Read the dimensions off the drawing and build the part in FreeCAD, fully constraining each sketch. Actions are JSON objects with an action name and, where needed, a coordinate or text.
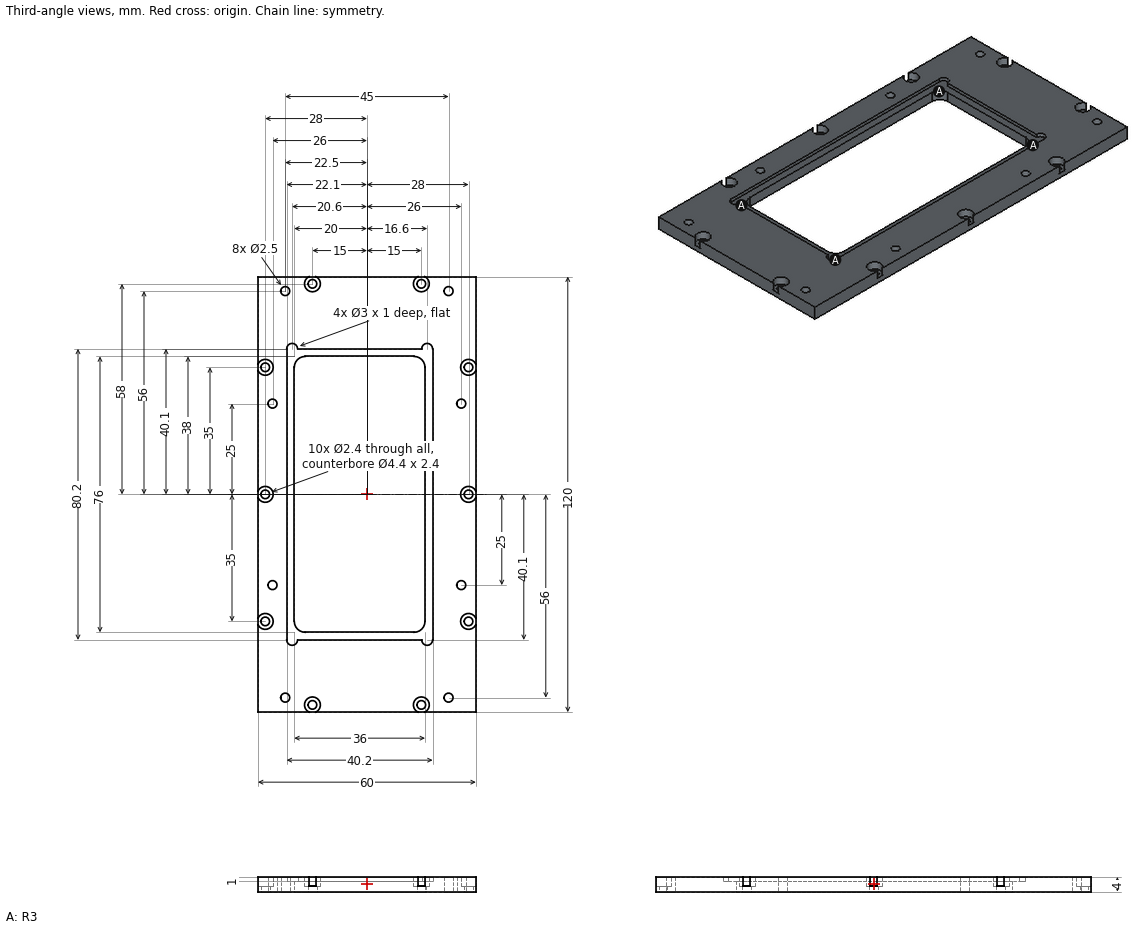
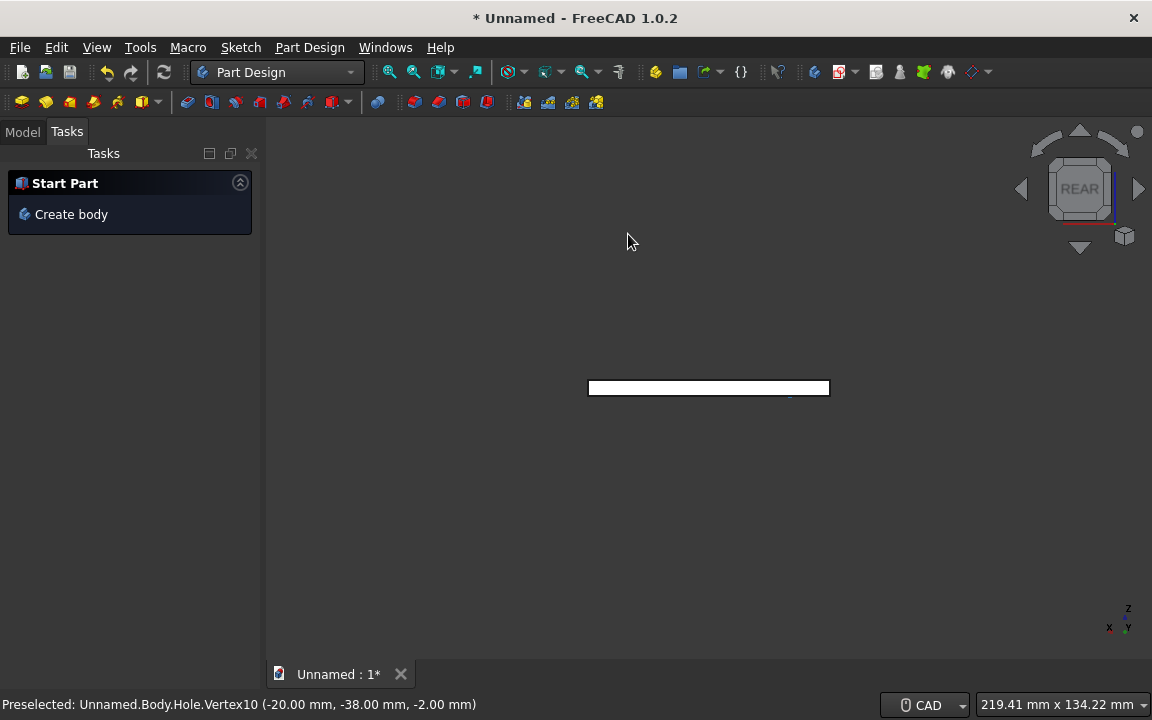
{"action": "key", "text": "v f"}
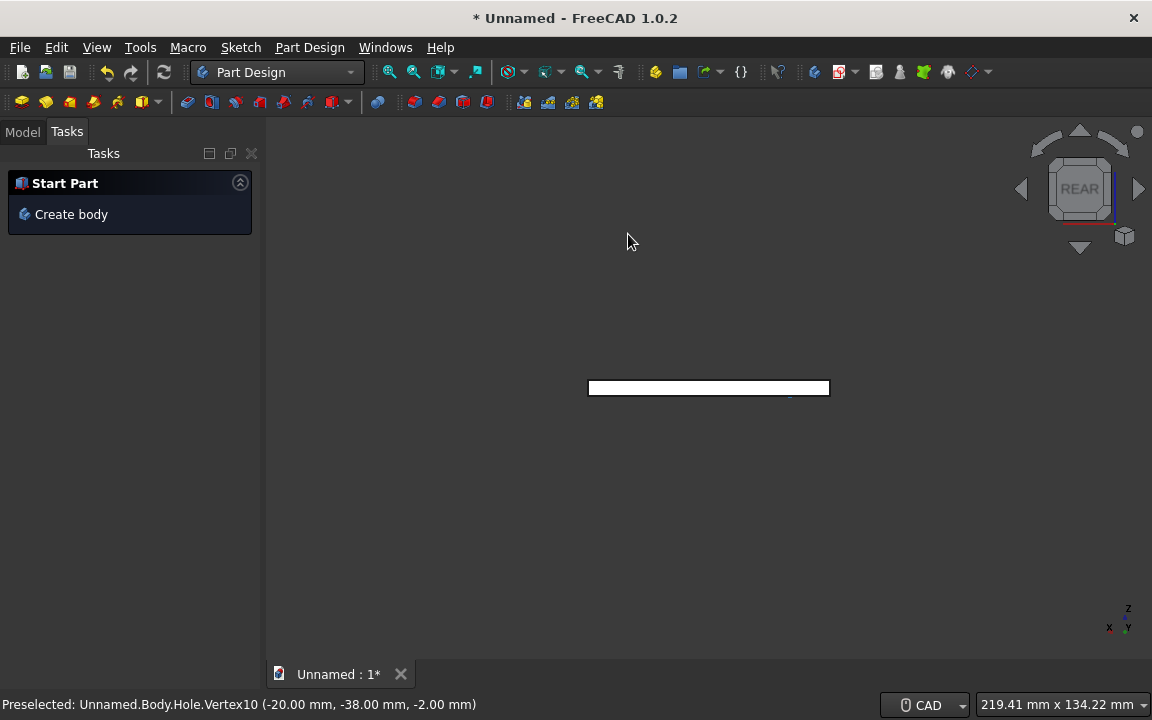
{"action": "scroll", "coordinate": [790, 389], "scroll_direction": "up", "scroll_amount": 6}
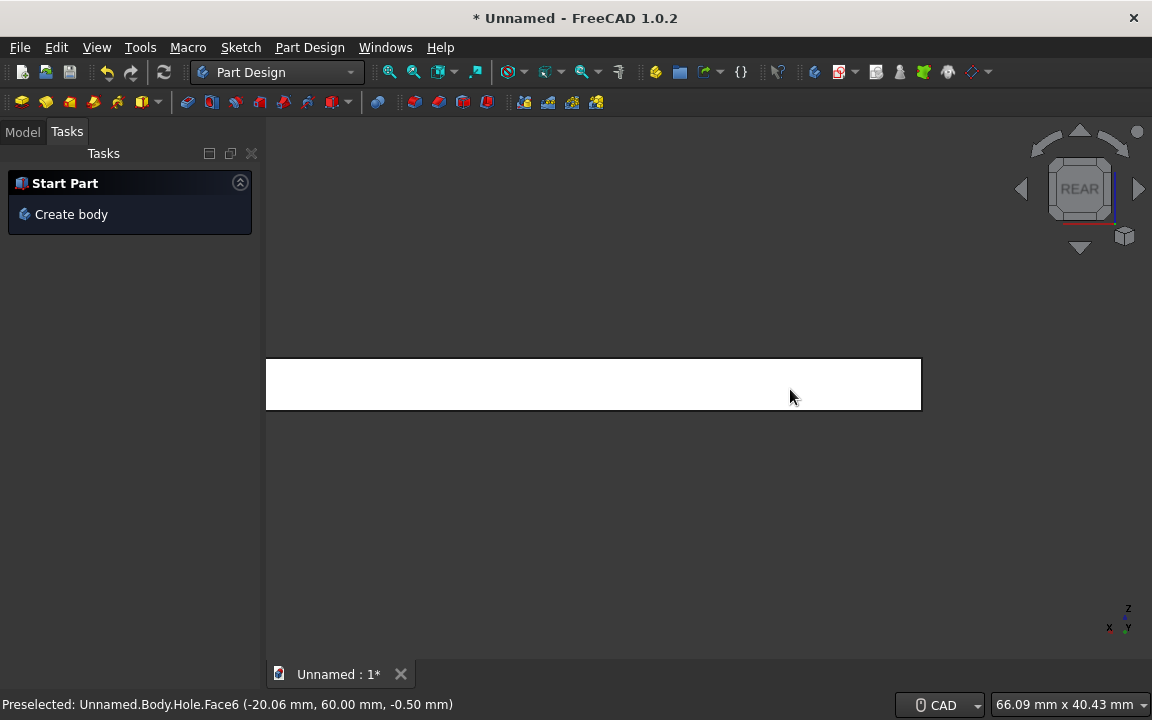
{"action": "key", "text": "v f"}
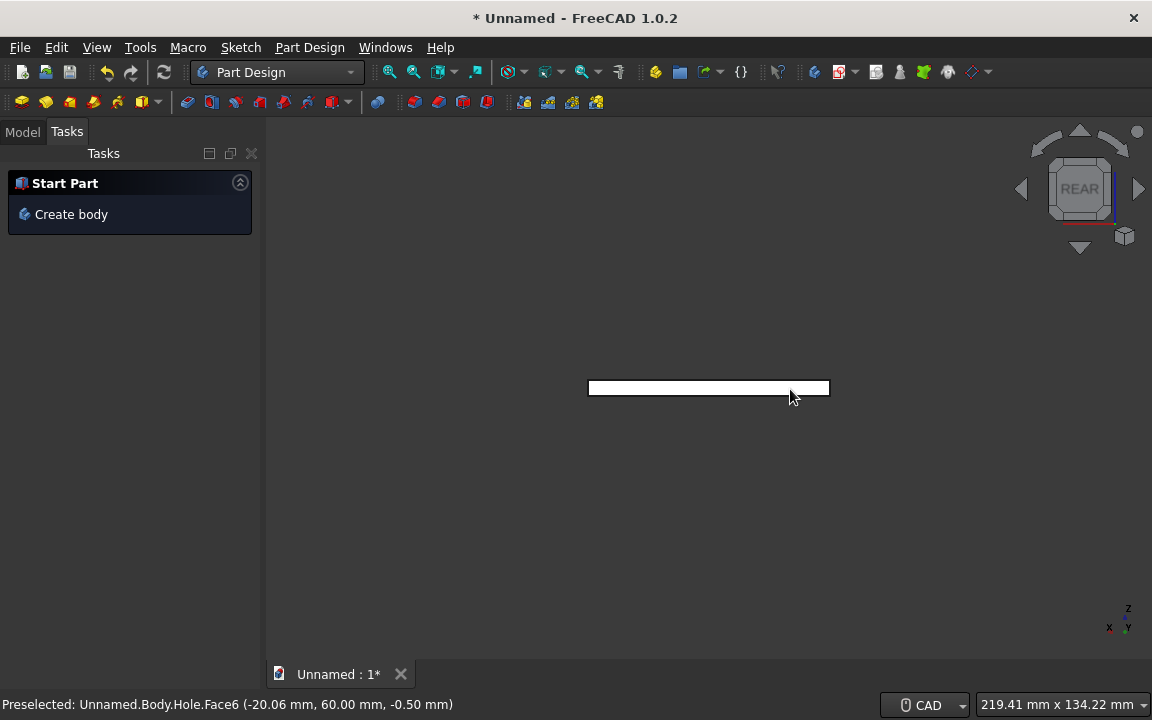
{"action": "key", "text": "6"}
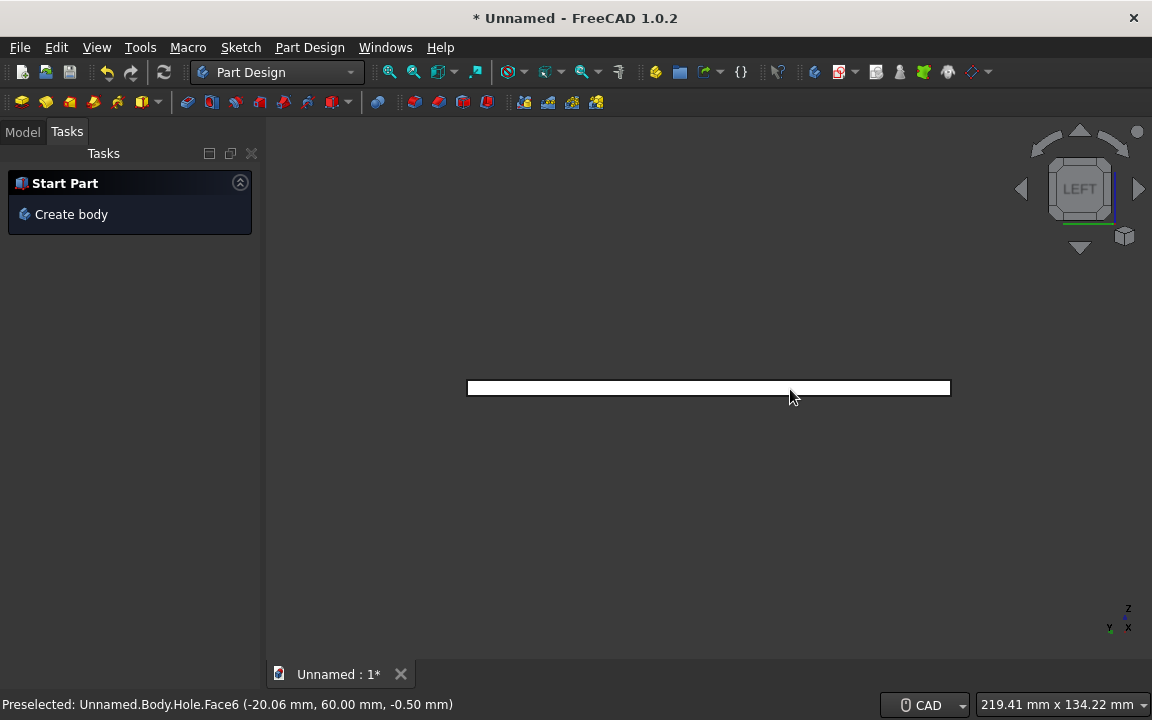
{"action": "scroll", "coordinate": [862, 389], "scroll_direction": "up", "scroll_amount": 6}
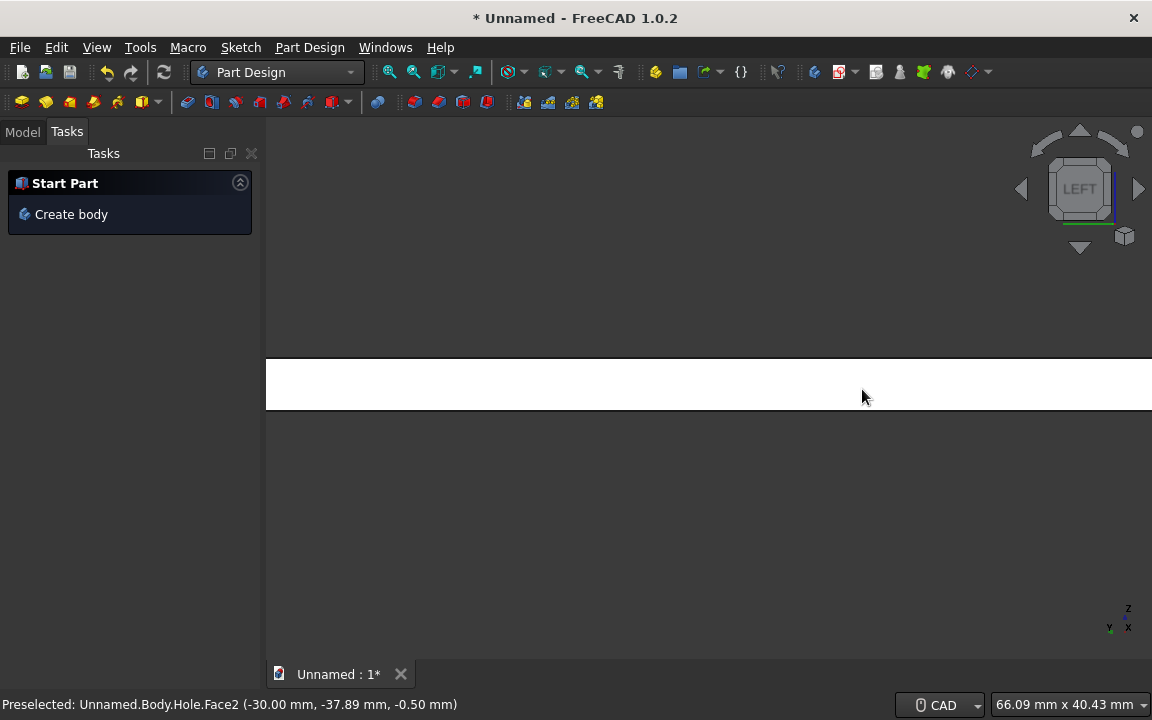
{"action": "key", "text": "v f"}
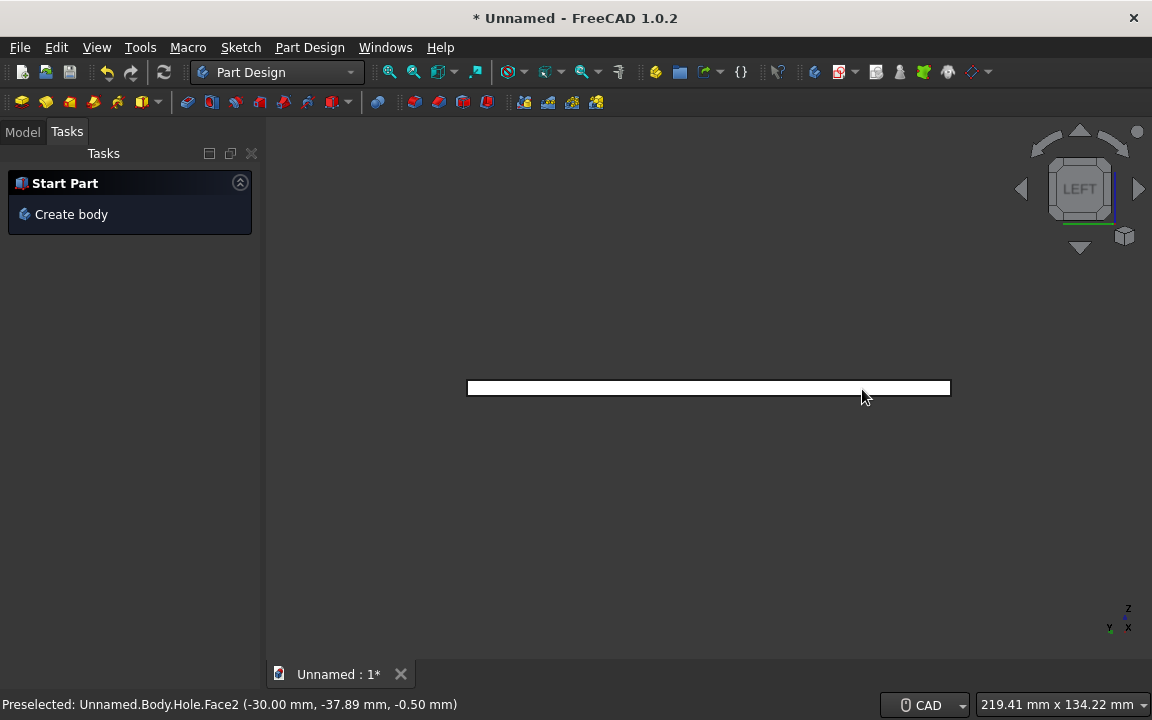
{"action": "key", "text": "v 3"}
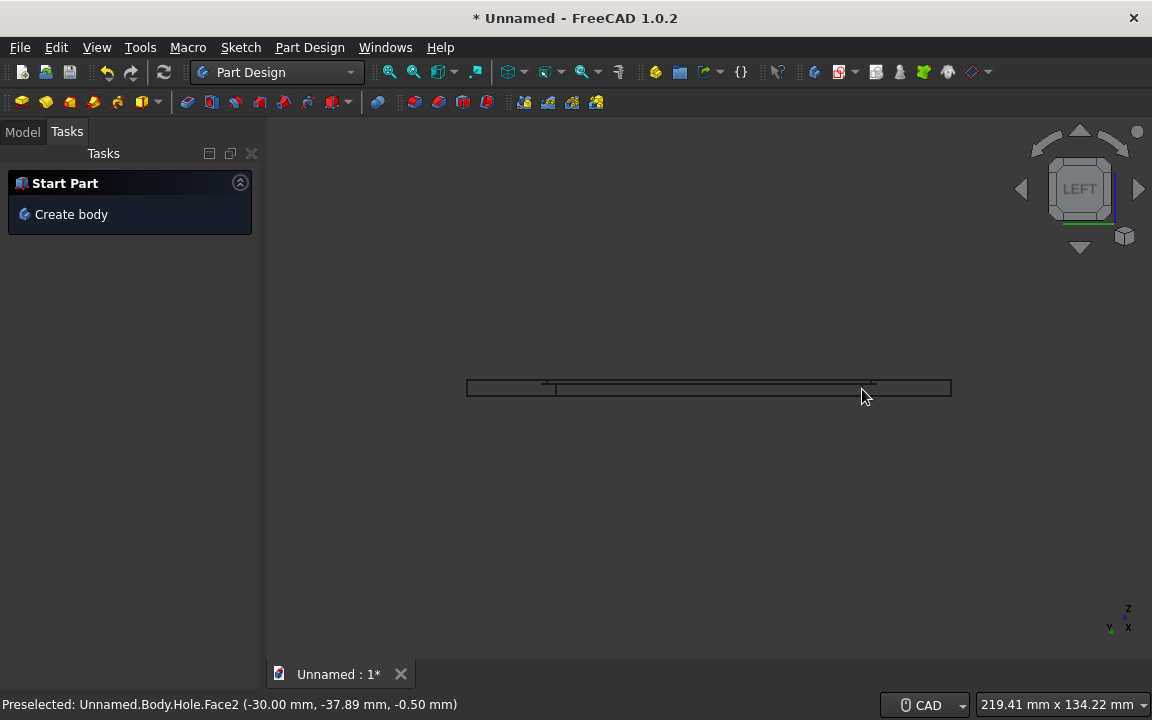
{"action": "key", "text": "0"}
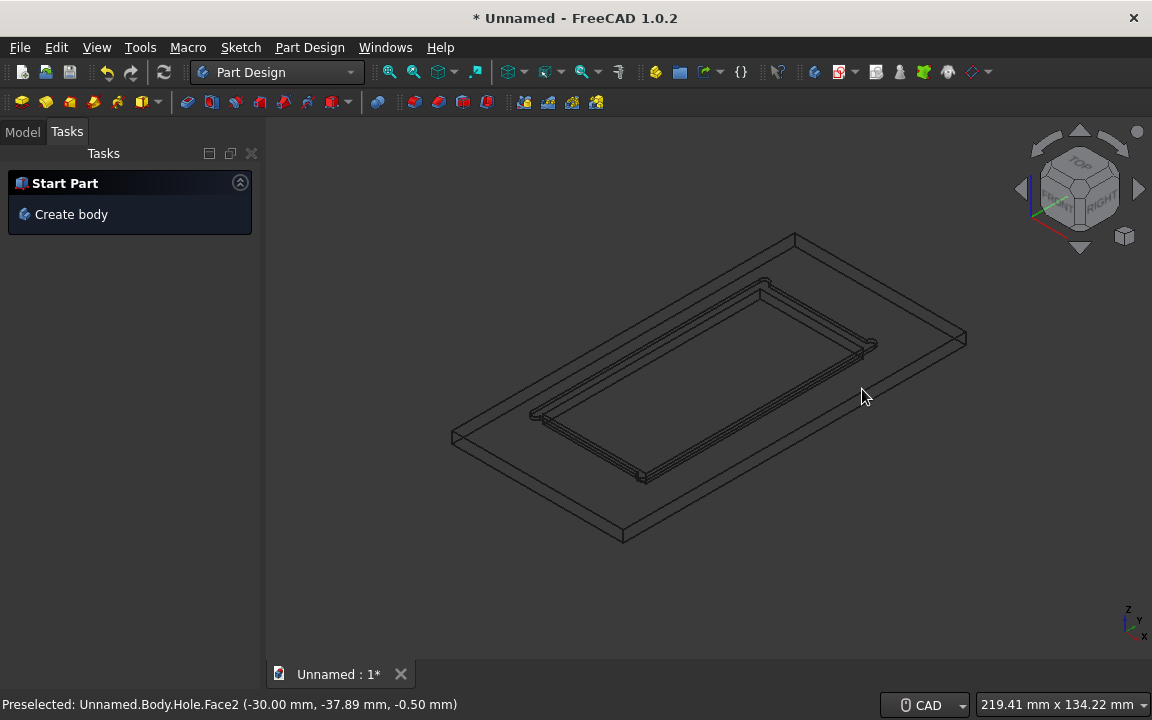
{"action": "left_click", "coordinate": [760, 296]}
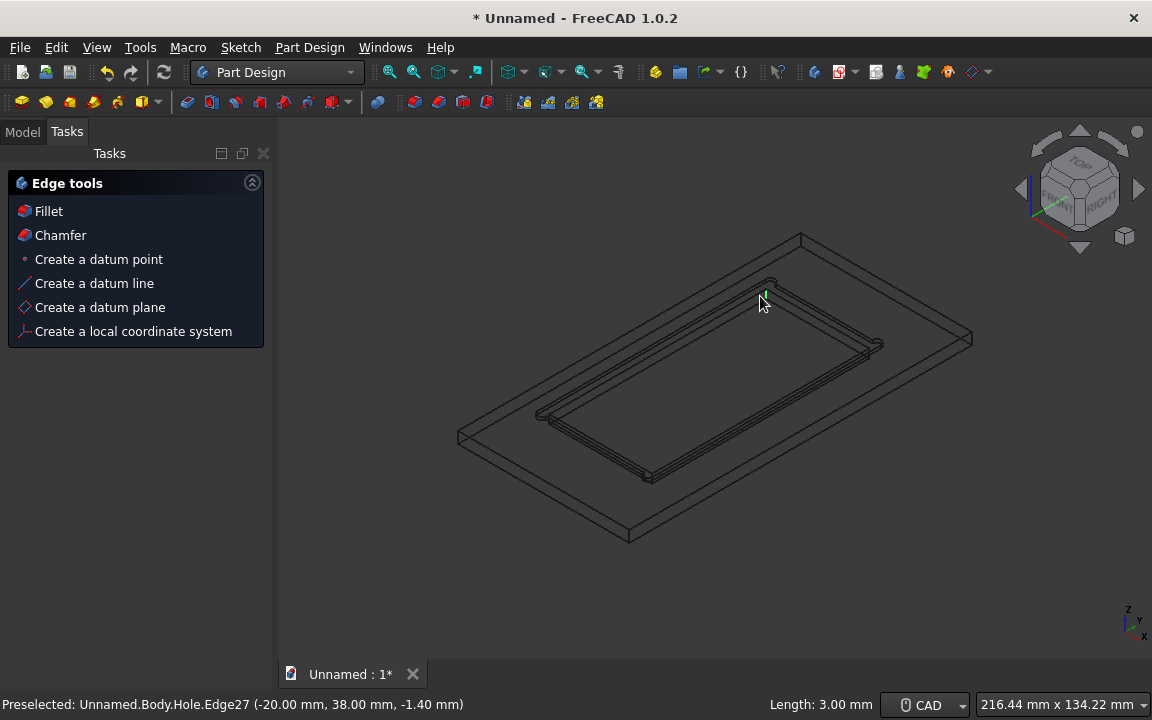
{"action": "scroll", "coordinate": [549, 418], "scroll_direction": "up", "scroll_amount": 6}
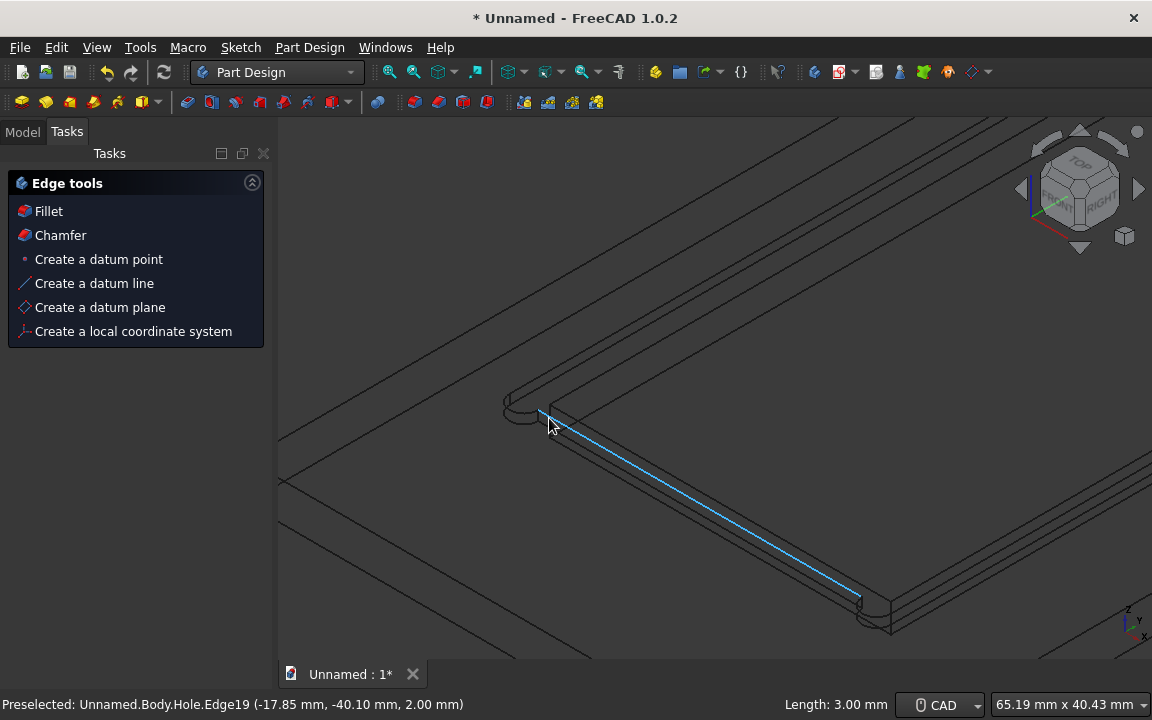
{"action": "key", "text": "v f"}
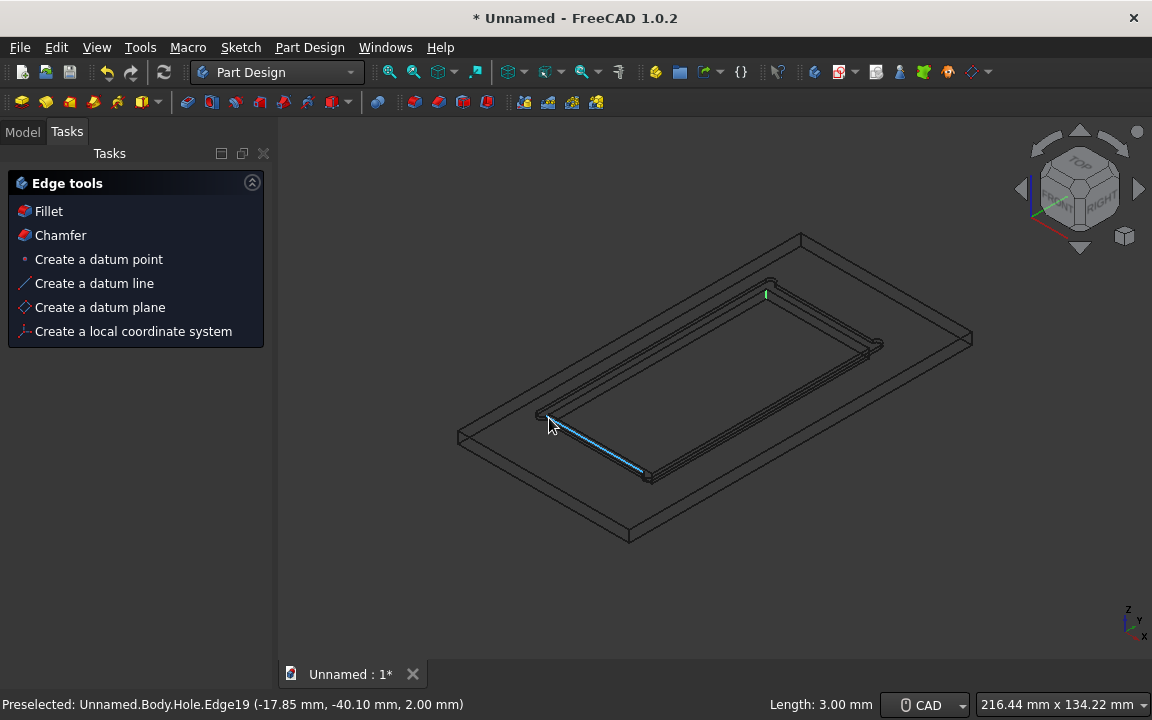
{"action": "key", "text": "2"}